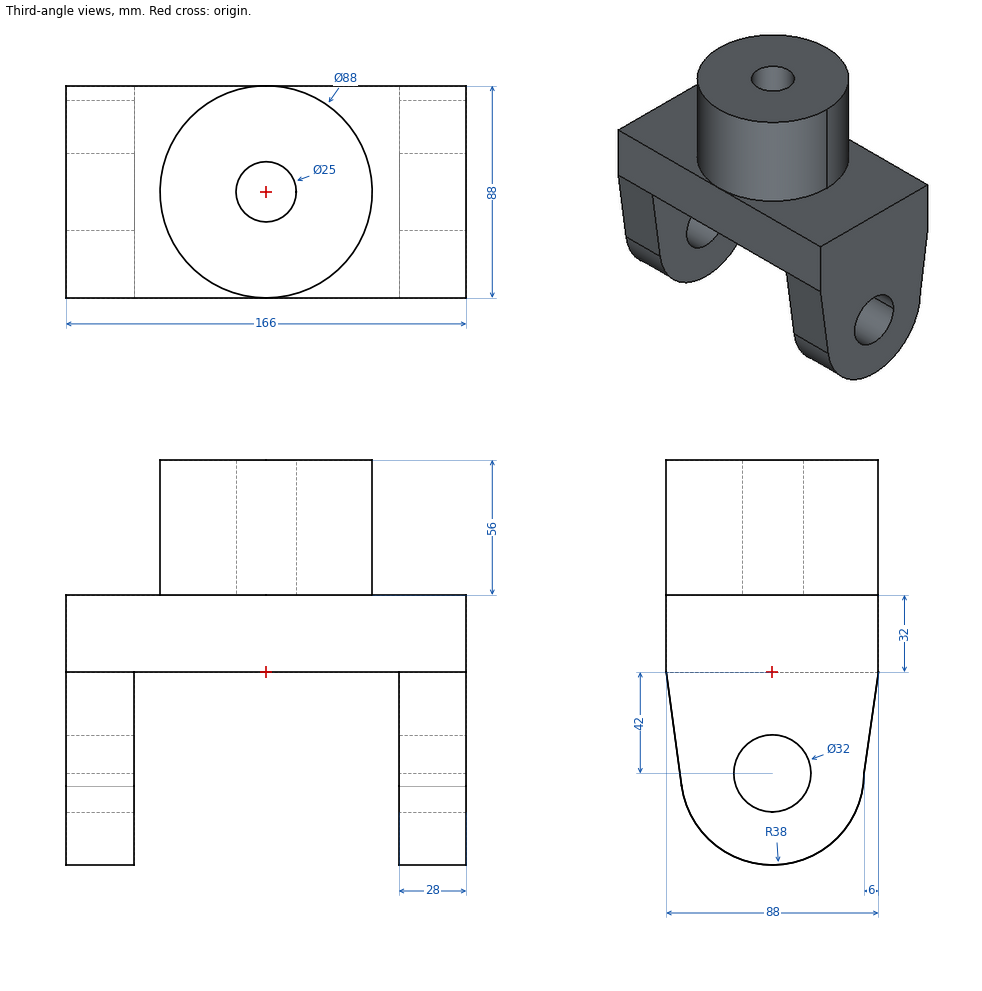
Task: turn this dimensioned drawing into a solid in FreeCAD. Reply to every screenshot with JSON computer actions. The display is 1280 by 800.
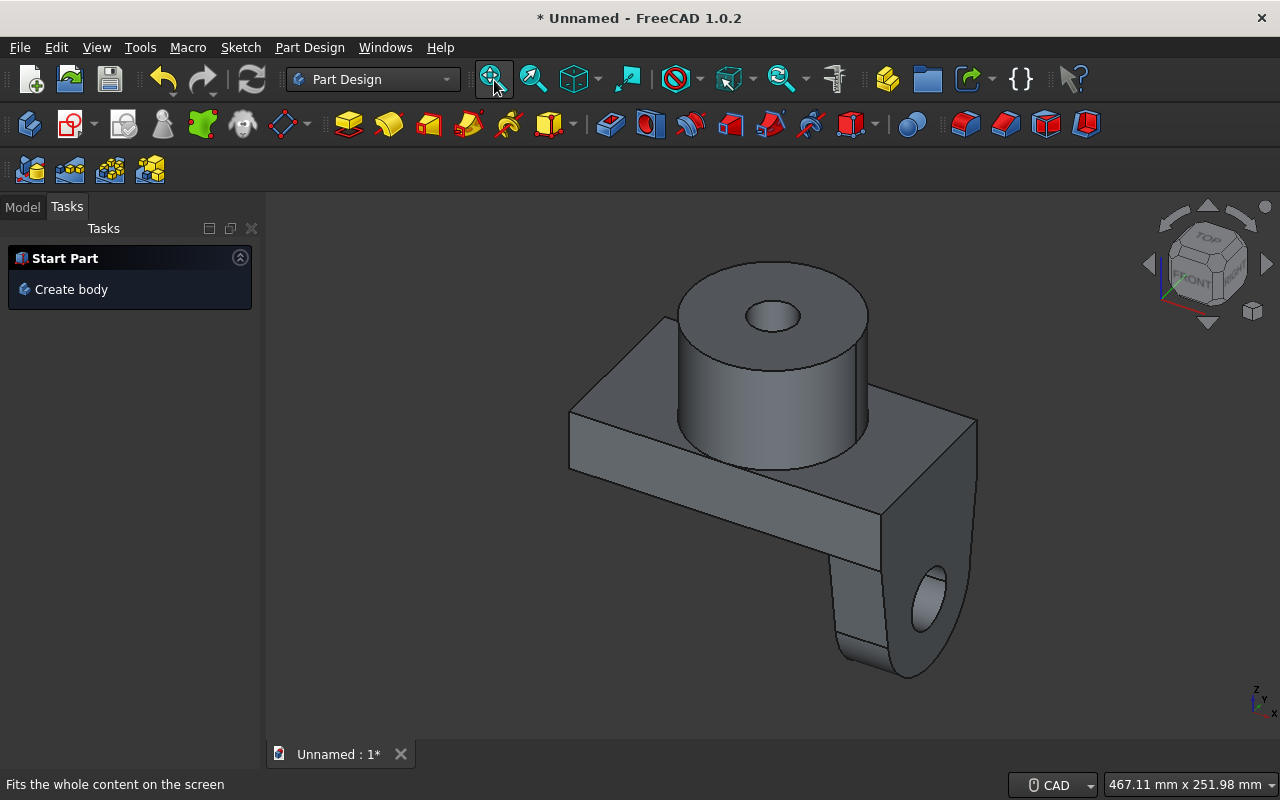
{"action": "left_click", "coordinate": [23, 206]}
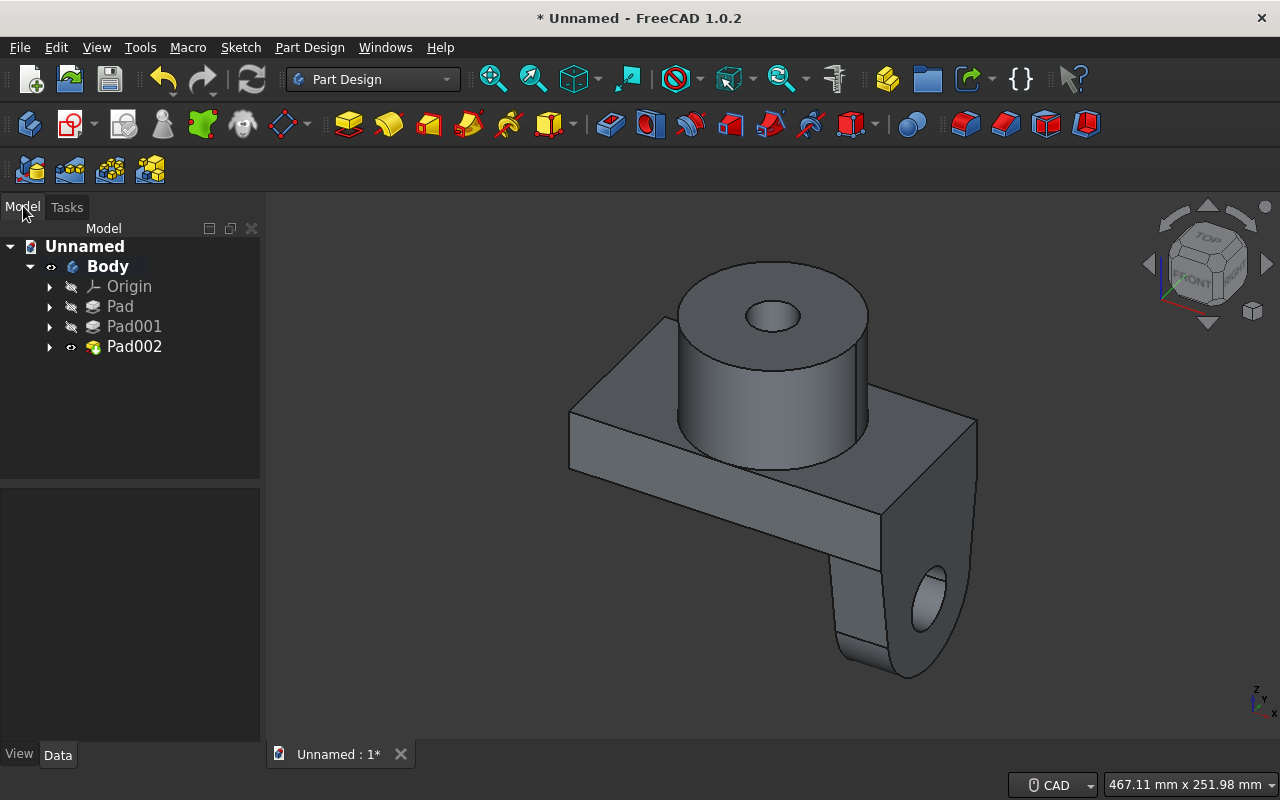
{"action": "left_click", "coordinate": [116, 347]}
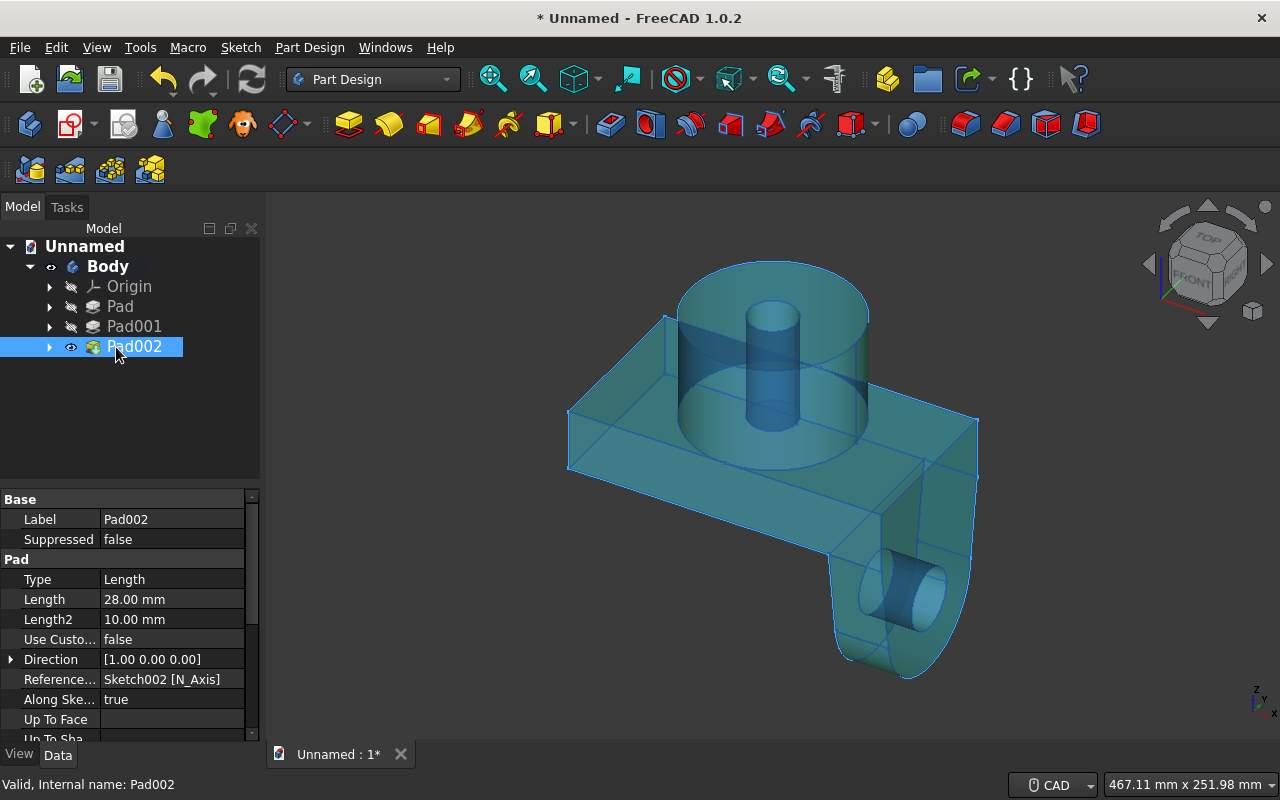
{"action": "left_click", "coordinate": [30, 170]}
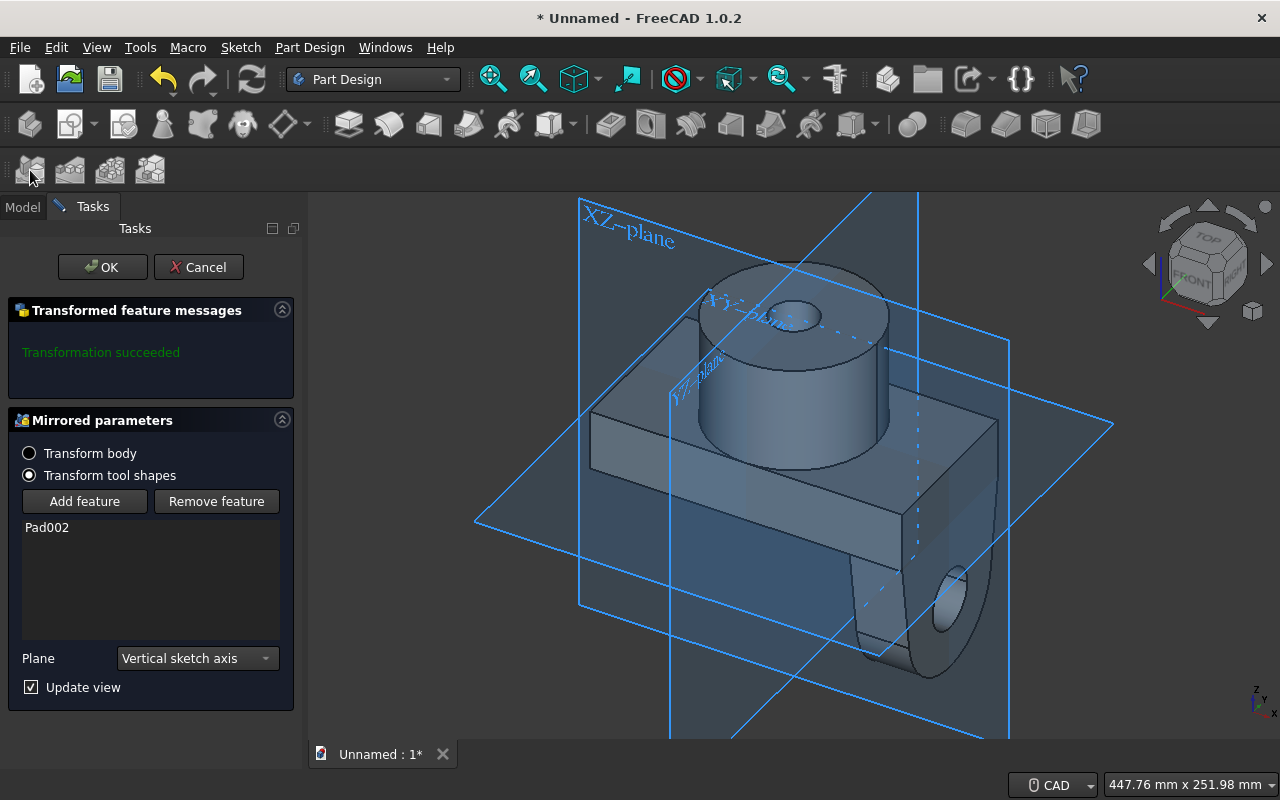
{"action": "left_click", "coordinate": [198, 658]}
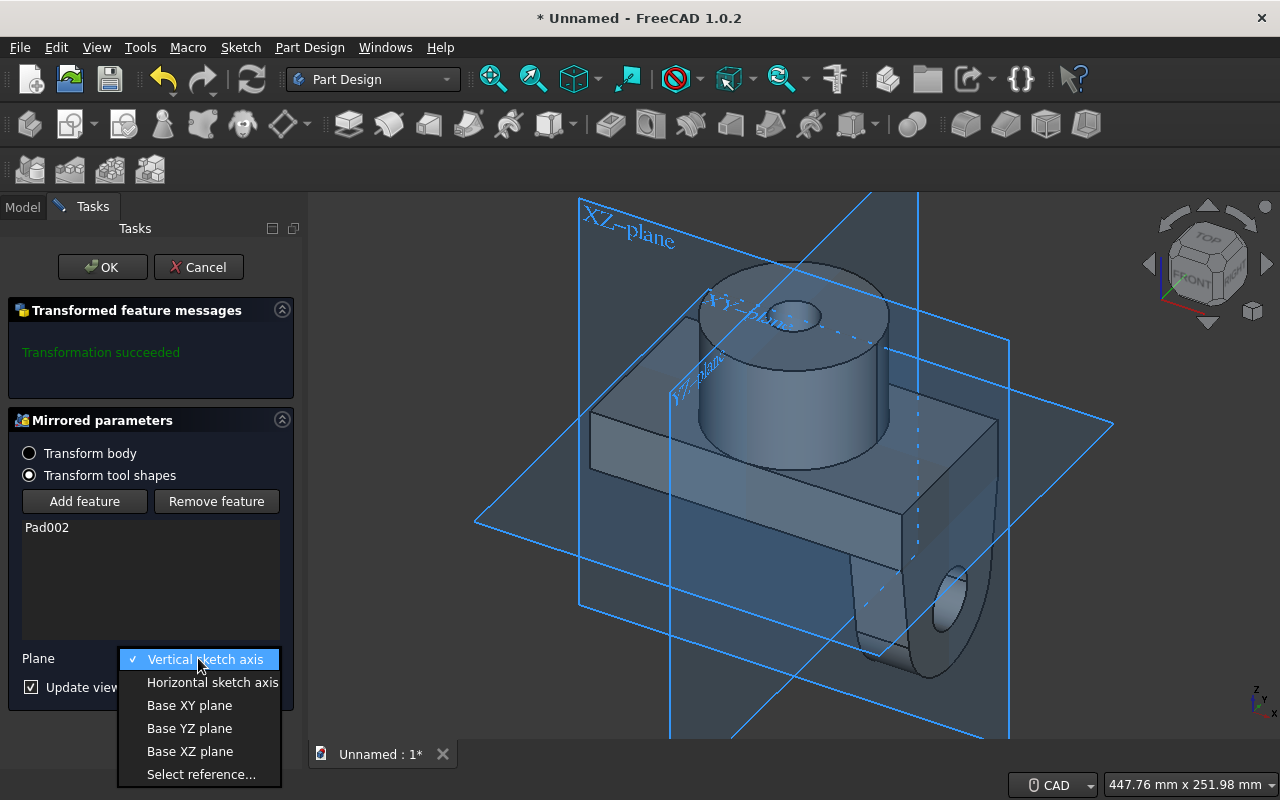
{"action": "left_click", "coordinate": [198, 728]}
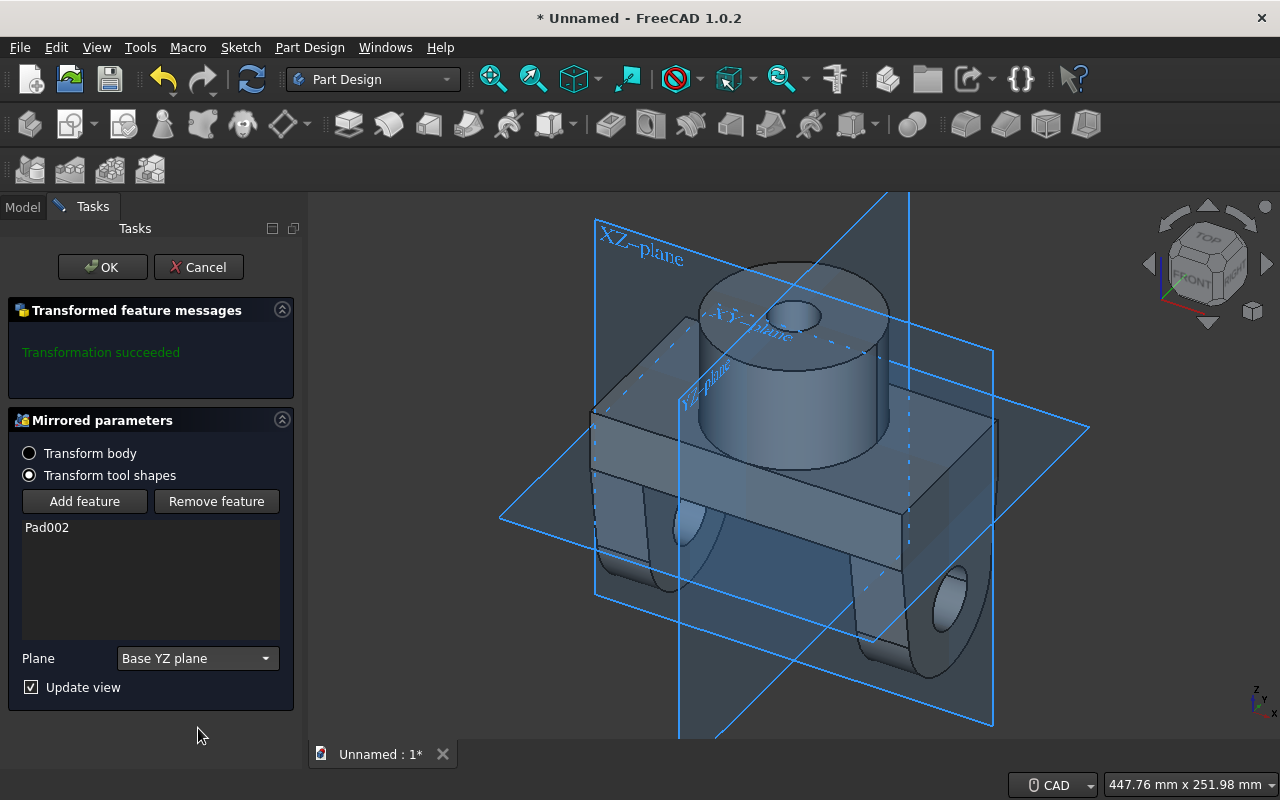
{"action": "left_click", "coordinate": [103, 267]}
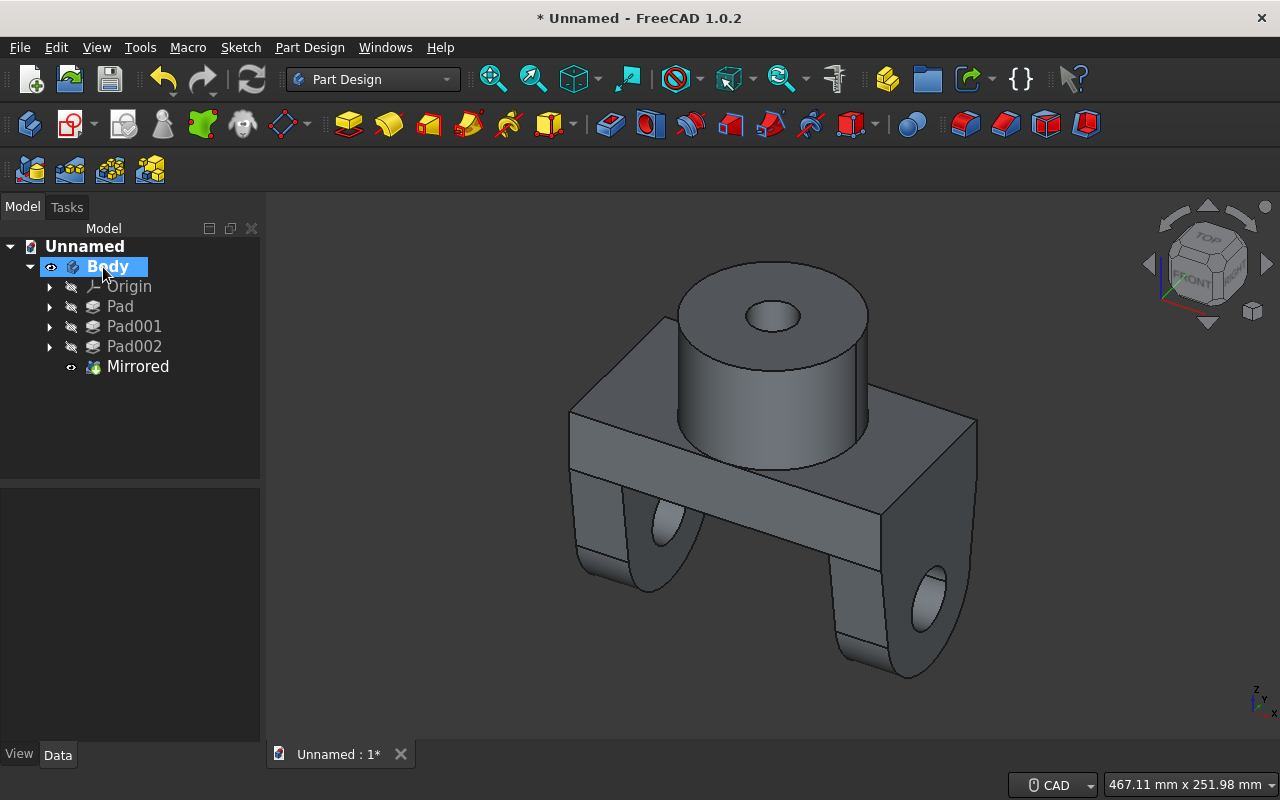
{"action": "key", "text": "0"}